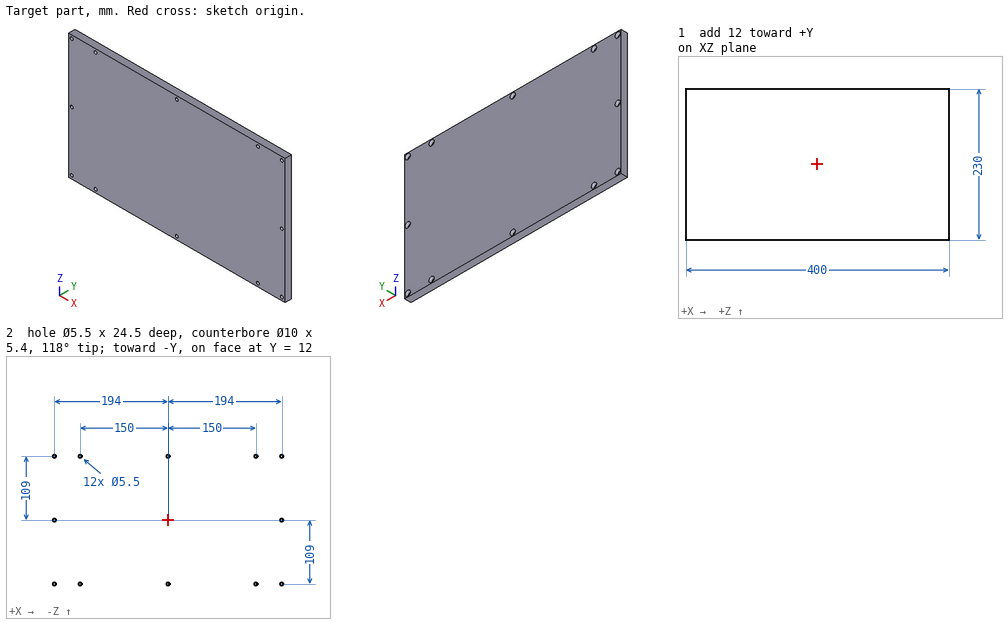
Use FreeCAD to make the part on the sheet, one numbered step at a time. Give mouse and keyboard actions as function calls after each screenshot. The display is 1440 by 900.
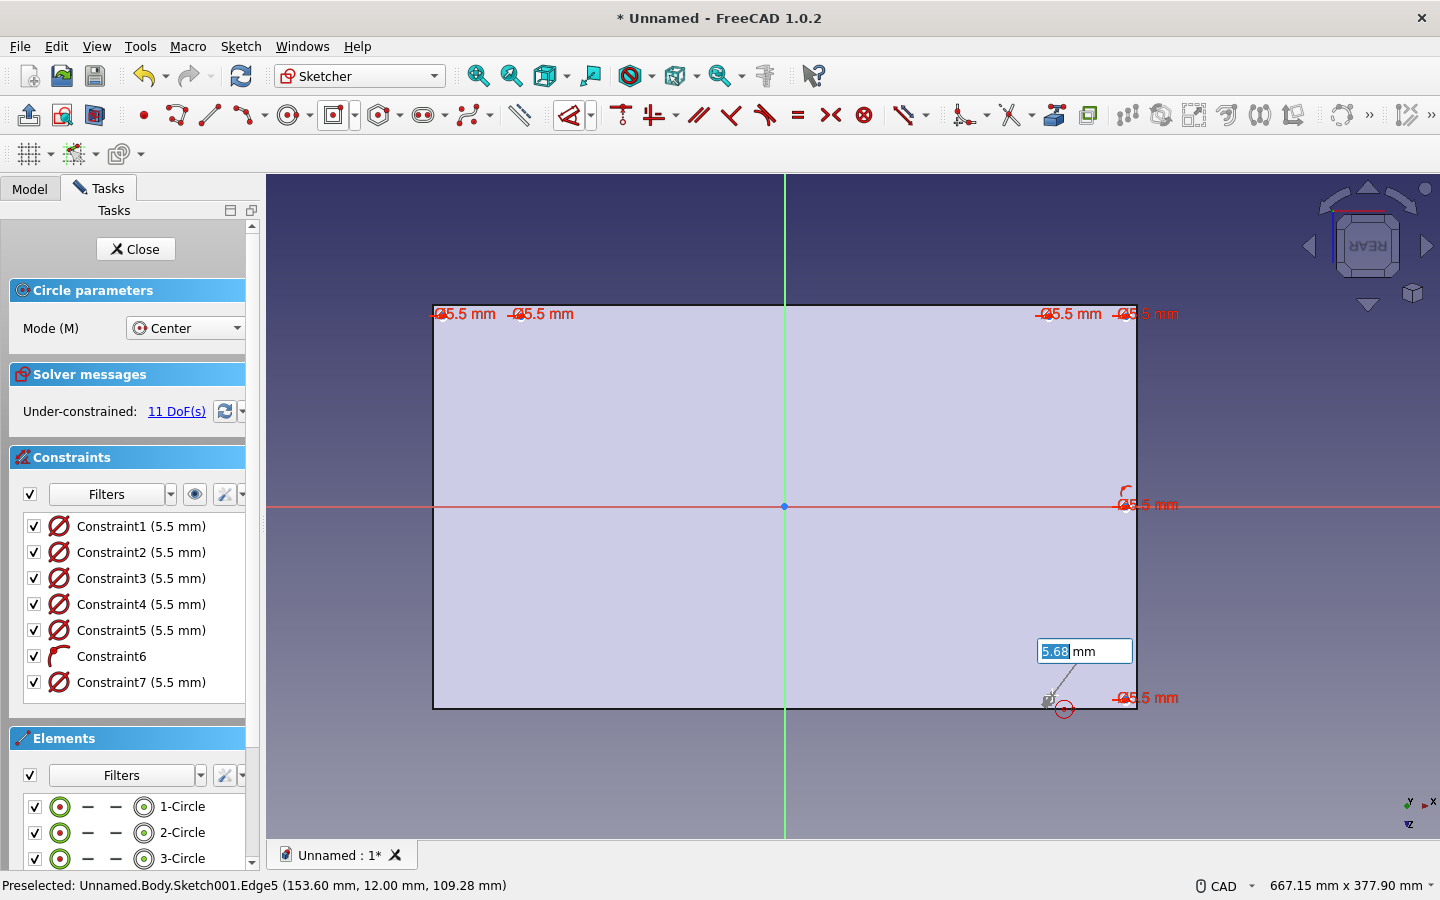
text(5.5)
key(Return)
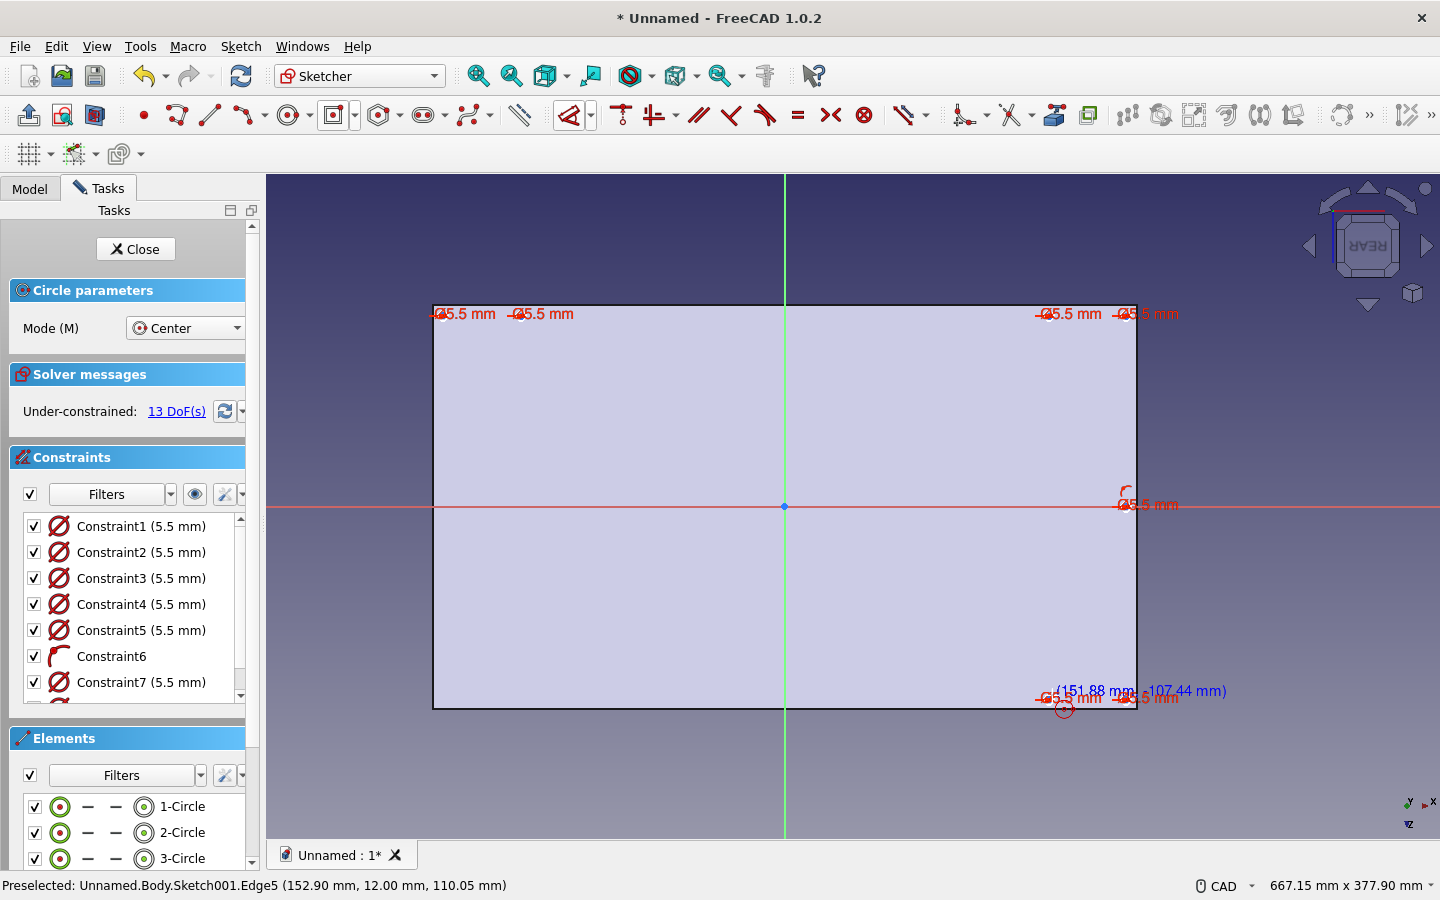
scroll(521, 699, up, 8)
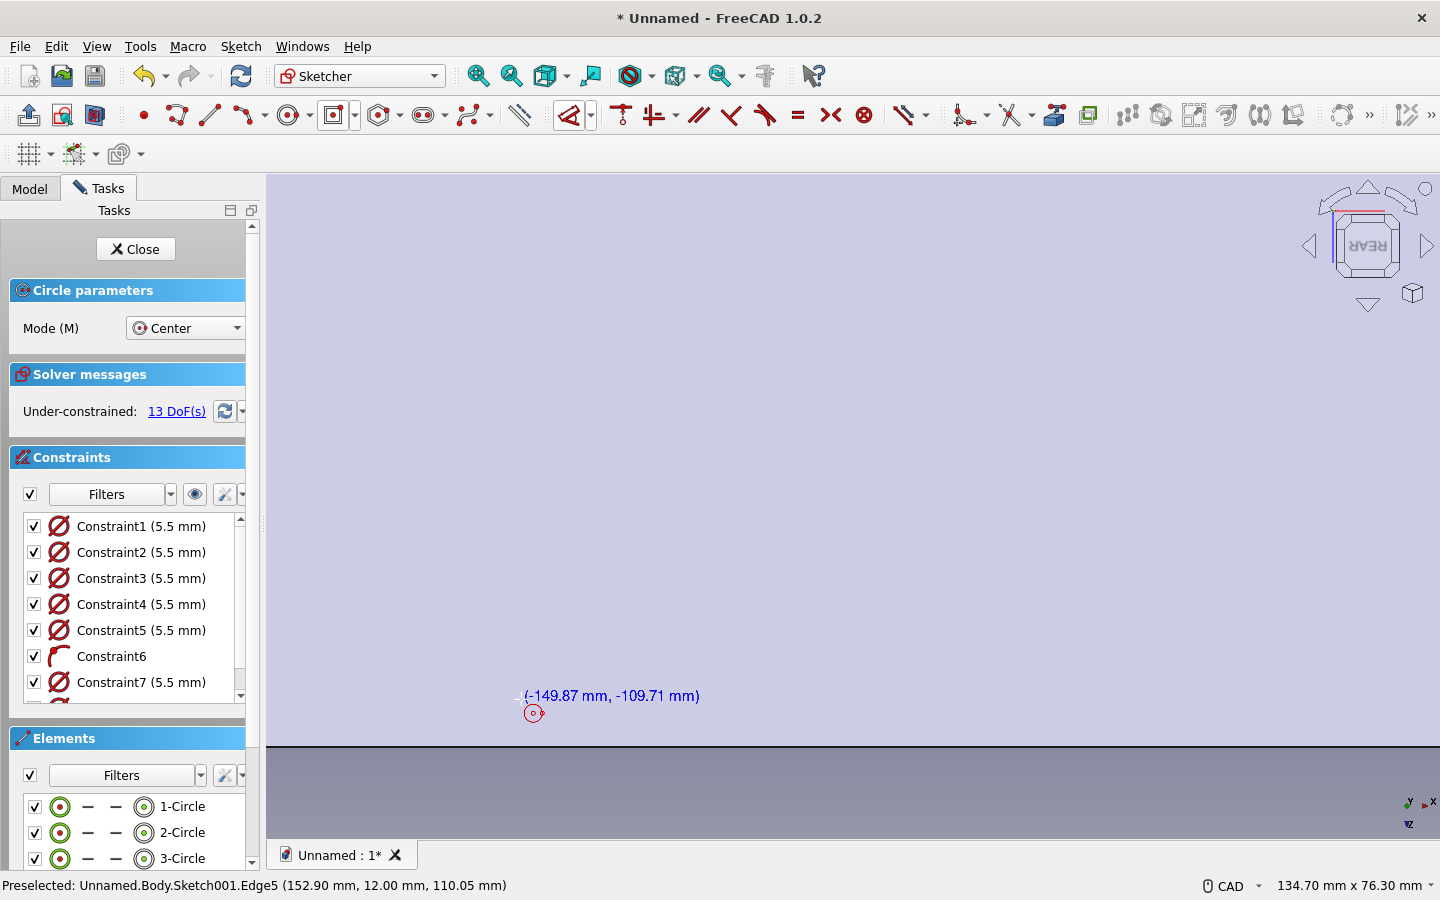
scroll(521, 699, down, 8)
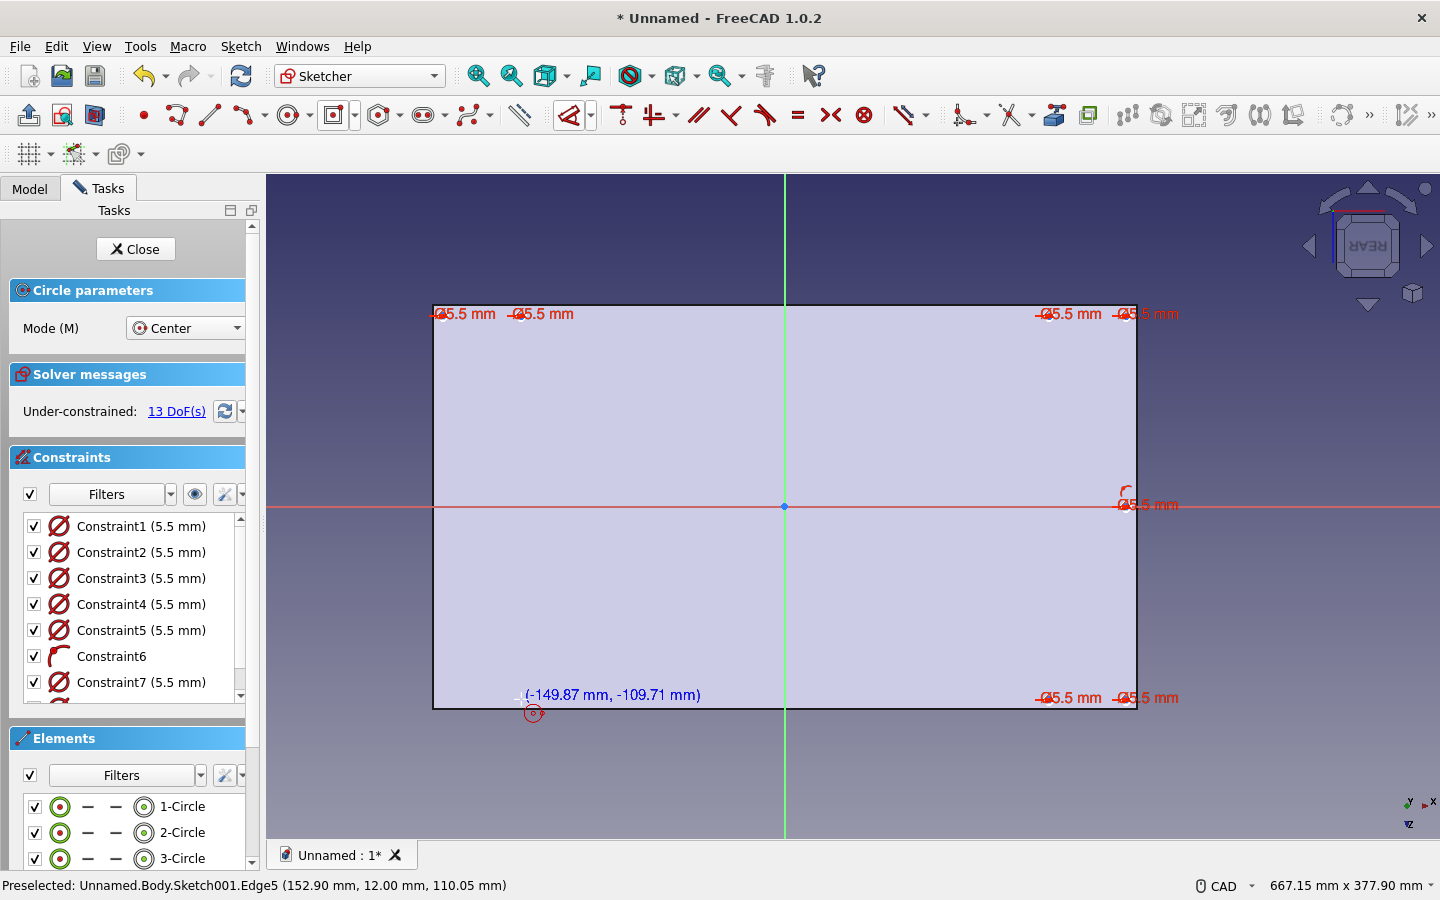
click(521, 699)
move(524, 695)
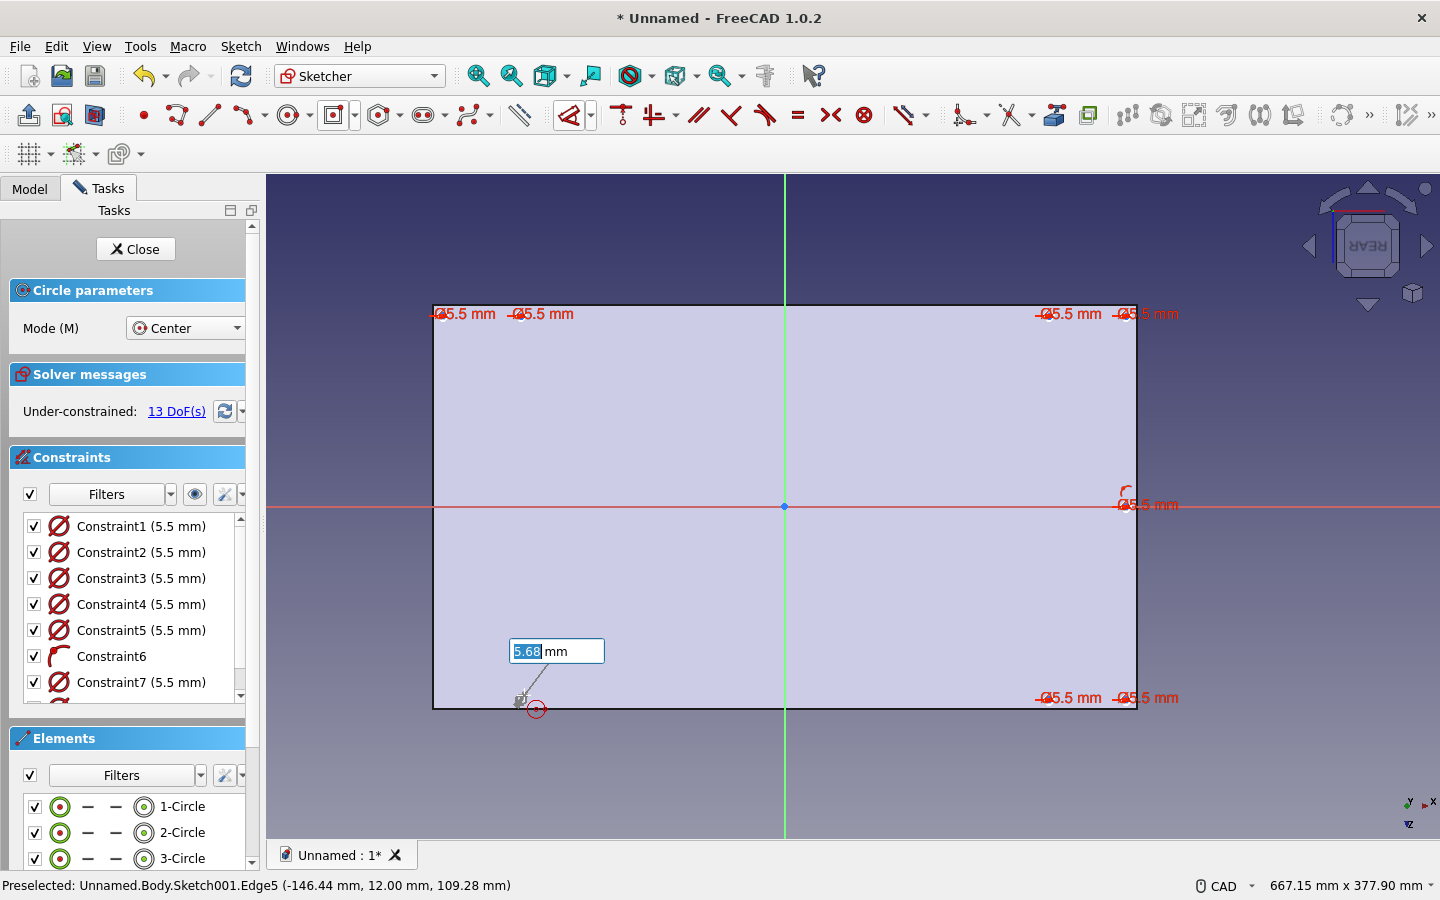
text(5.5)
key(Return)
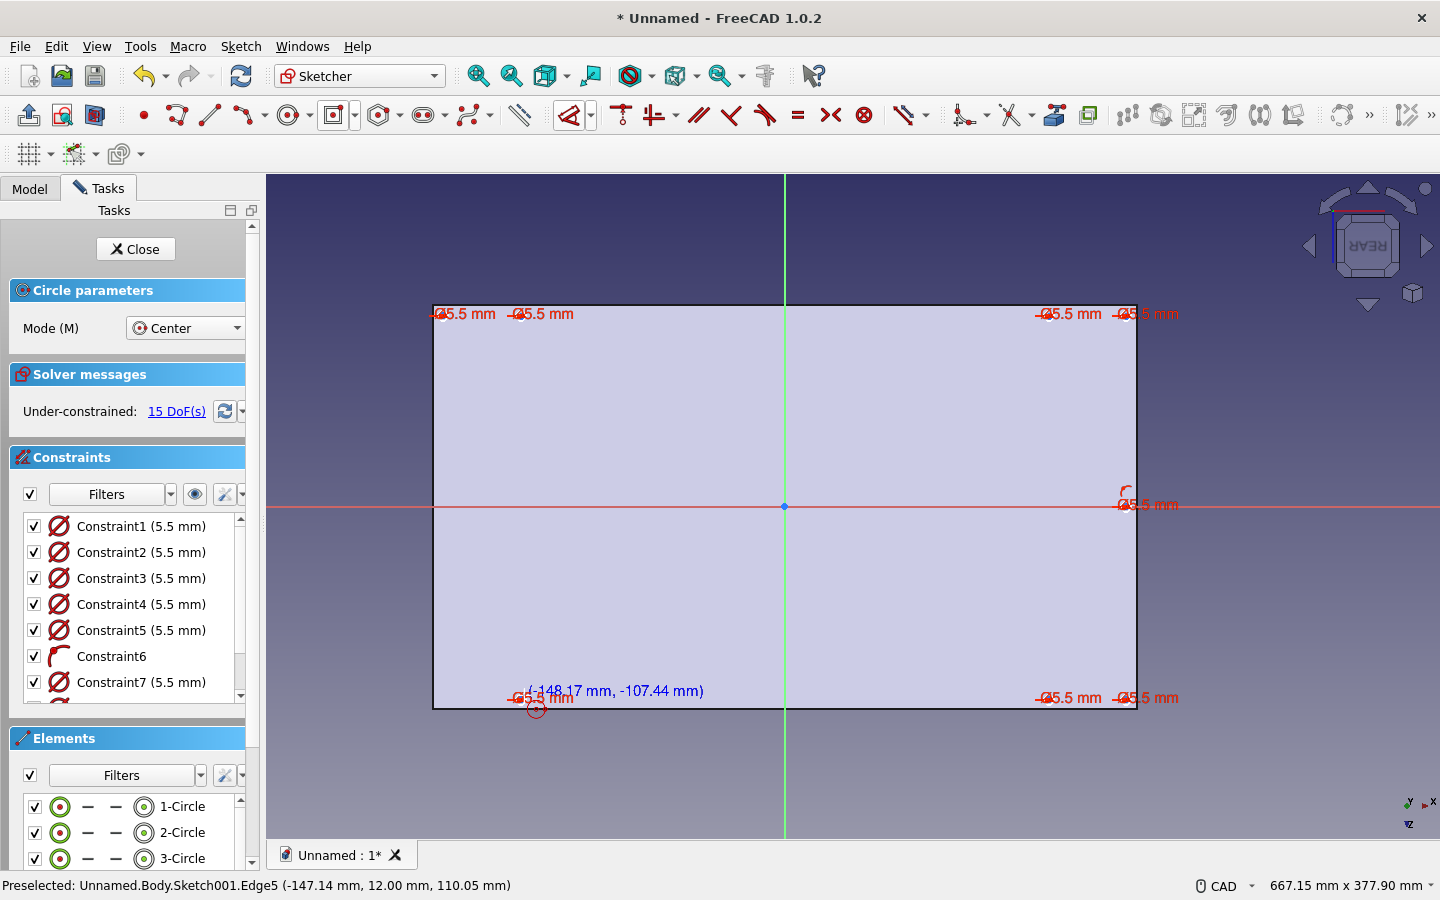
scroll(443, 699, up, 8)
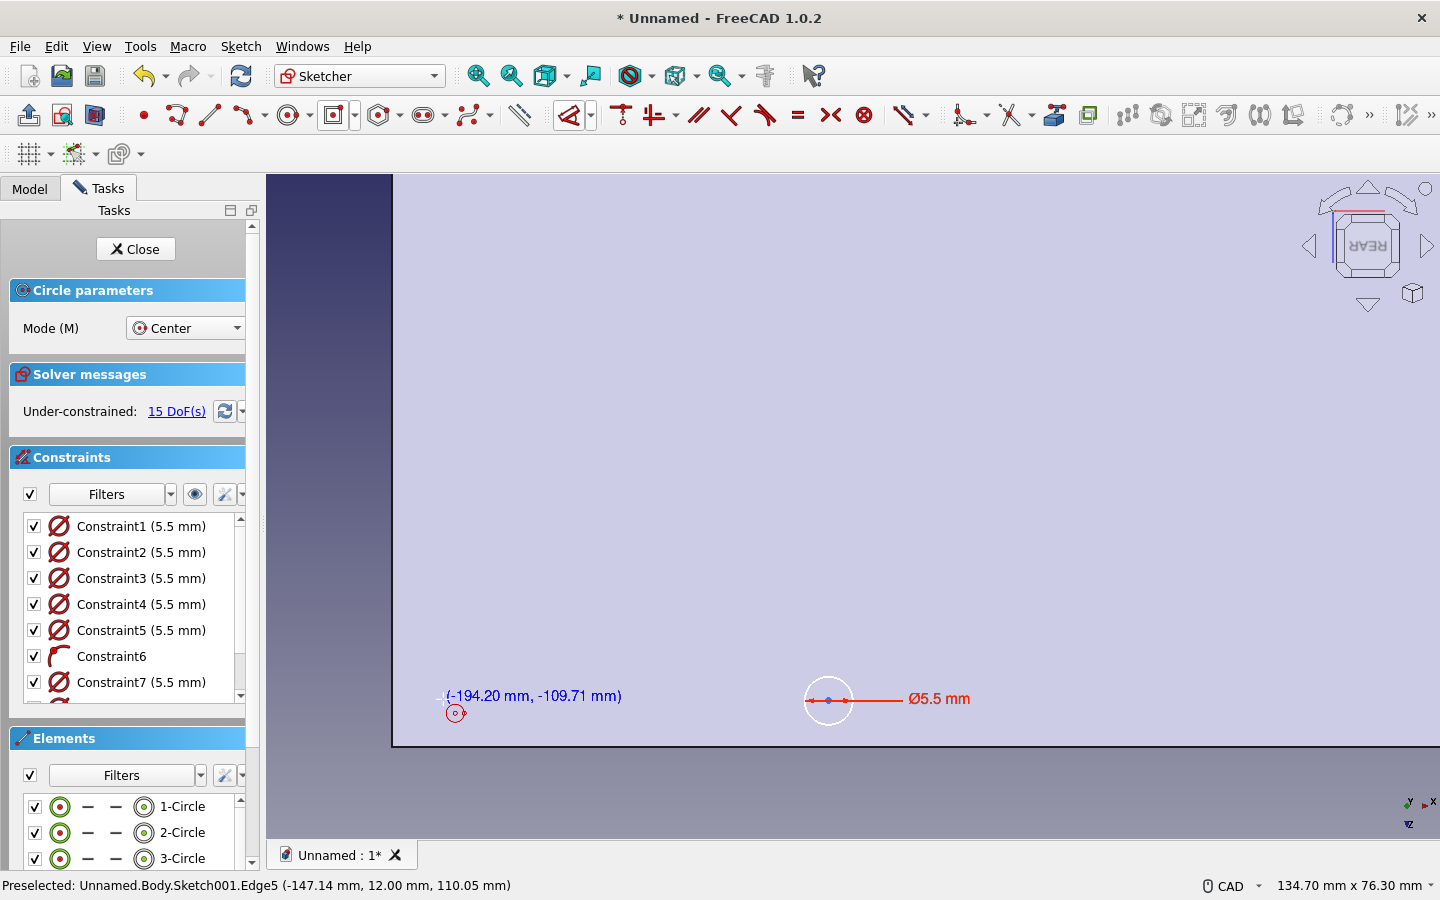
scroll(443, 699, down, 8)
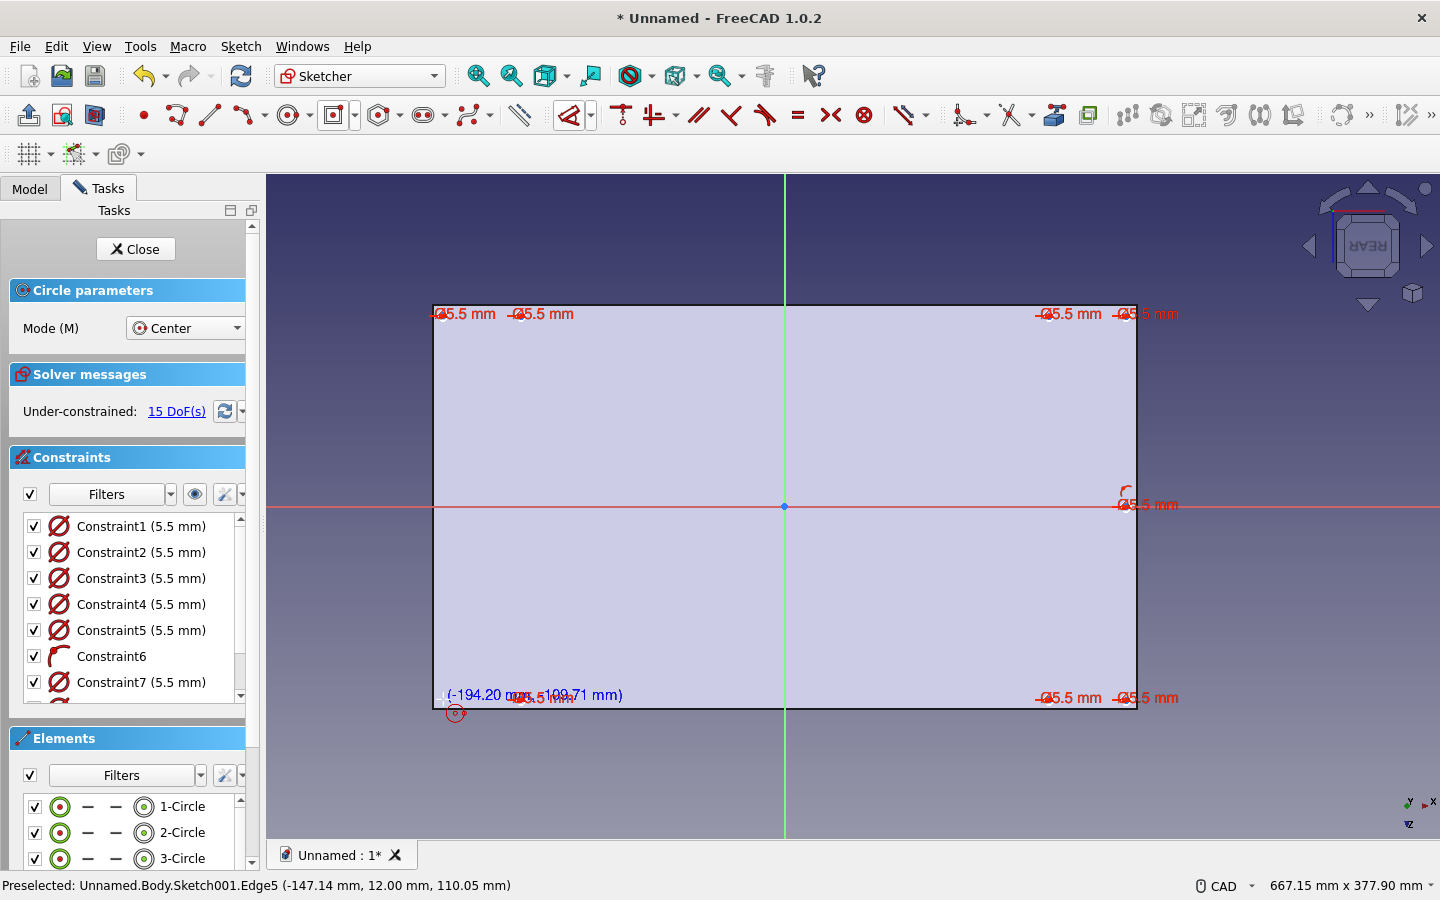
click(443, 699)
move(447, 695)